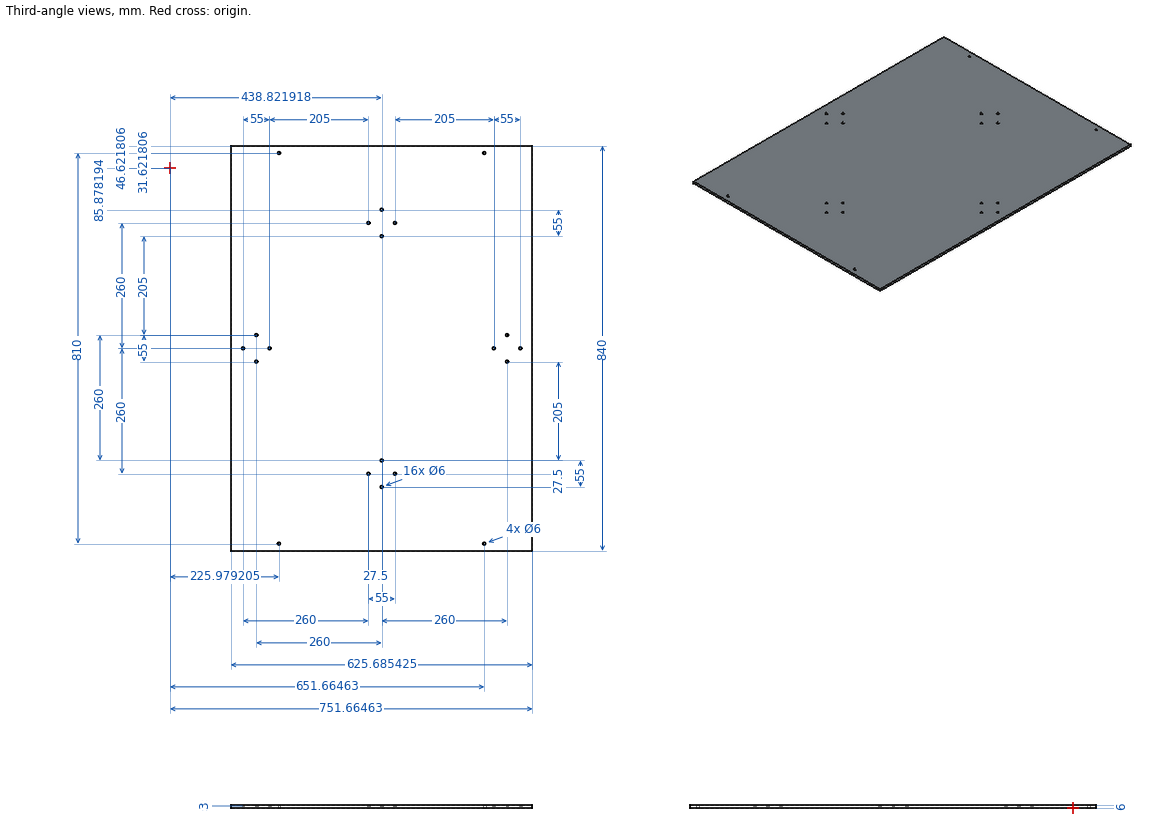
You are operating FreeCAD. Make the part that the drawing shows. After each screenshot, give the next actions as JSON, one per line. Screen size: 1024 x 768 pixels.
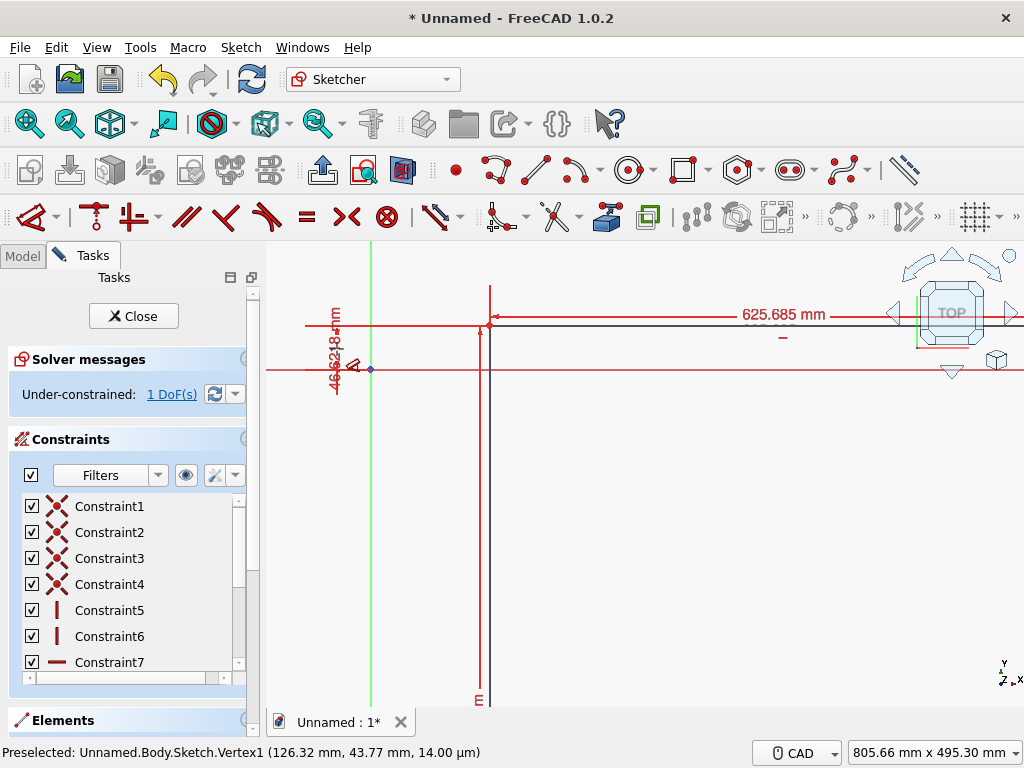
{"action": "scroll", "coordinate": [490, 330], "scroll_direction": "down", "scroll_amount": 5}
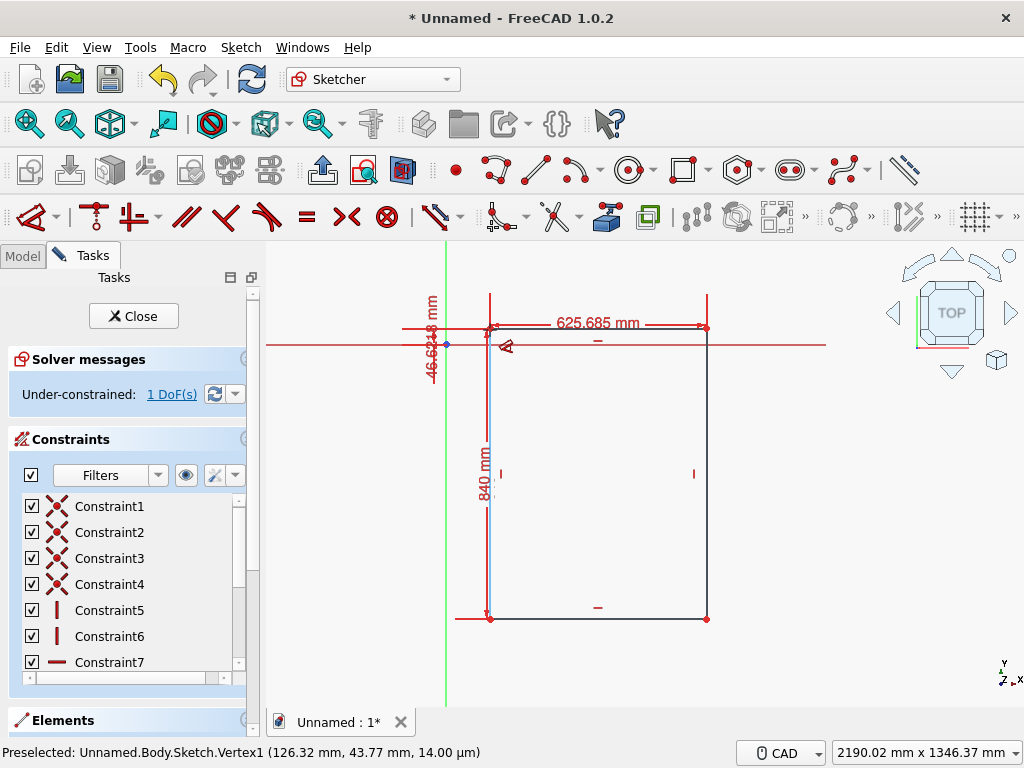
{"action": "left_click", "coordinate": [707, 619]}
{"action": "left_click", "coordinate": [576, 653]}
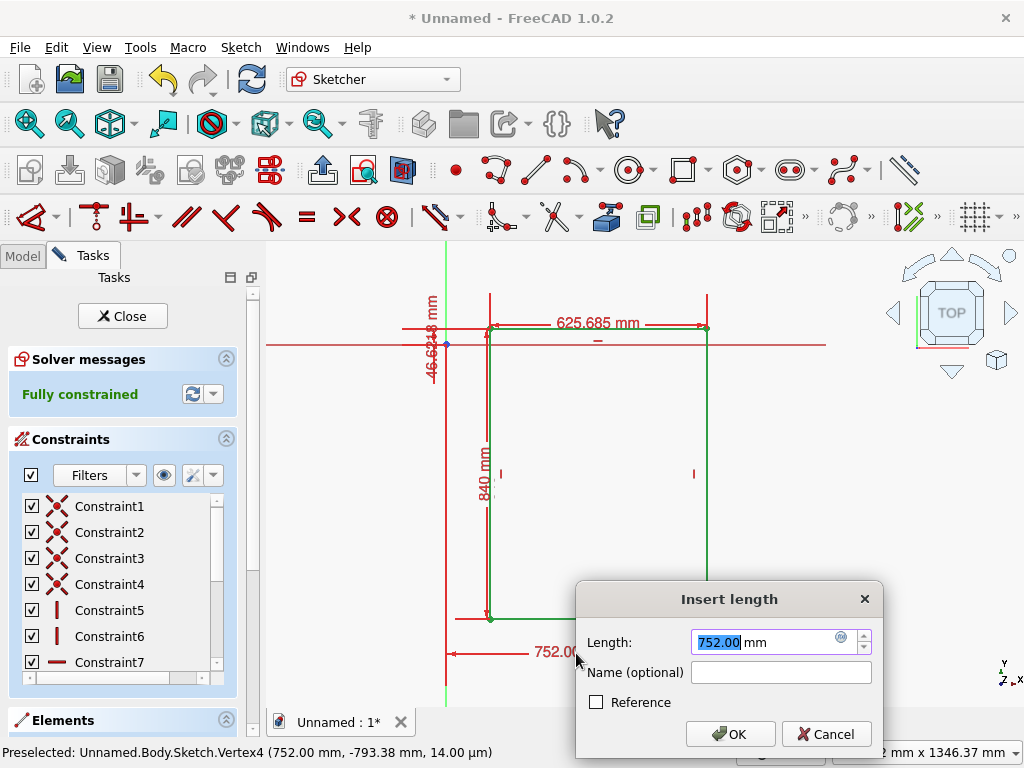
{"action": "type", "text": "751.66463"}
{"action": "key", "text": "Return"}
{"action": "key", "text": "Escape"}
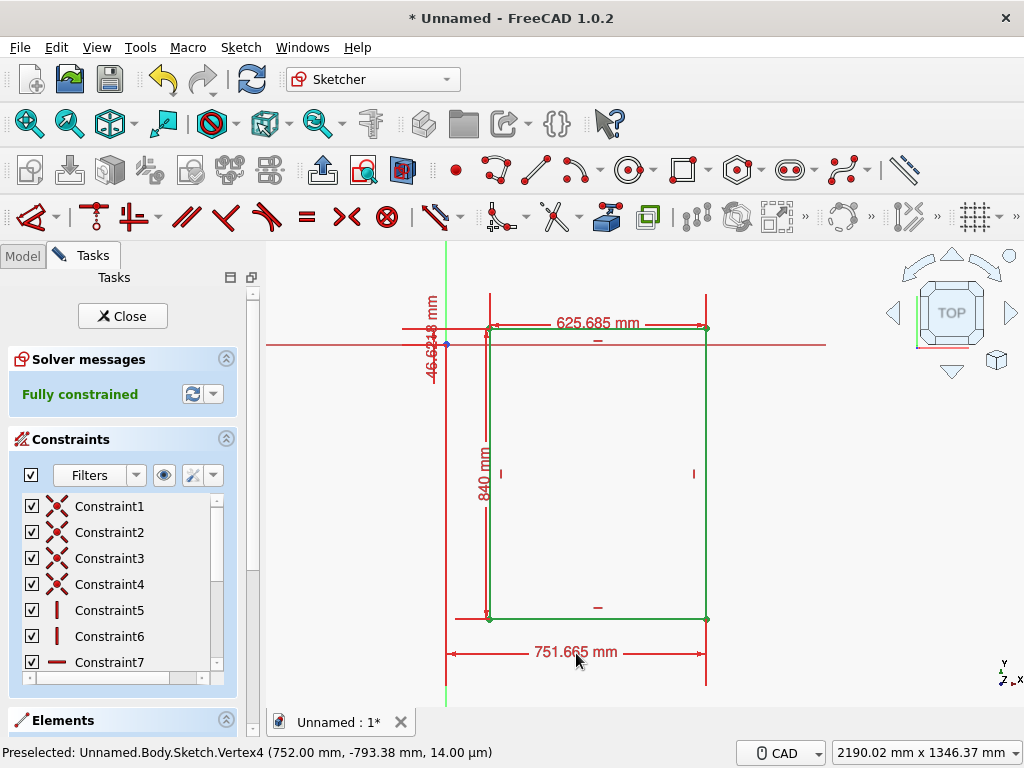
{"action": "left_click", "coordinate": [123, 316]}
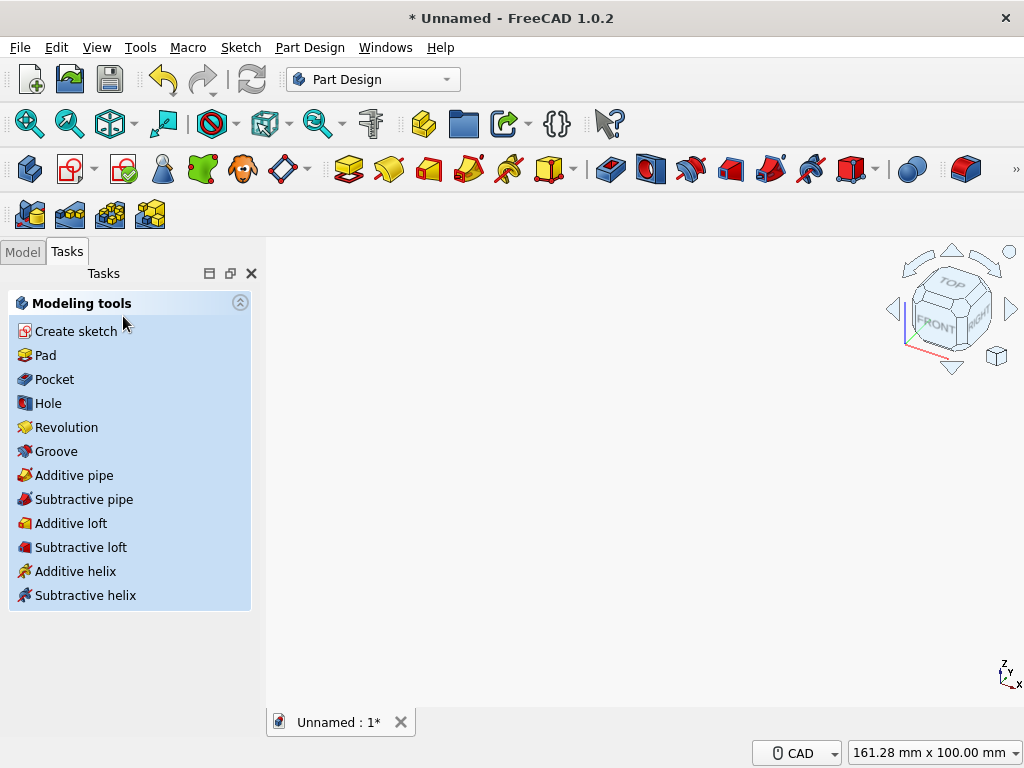
{"action": "left_click", "coordinate": [350, 170]}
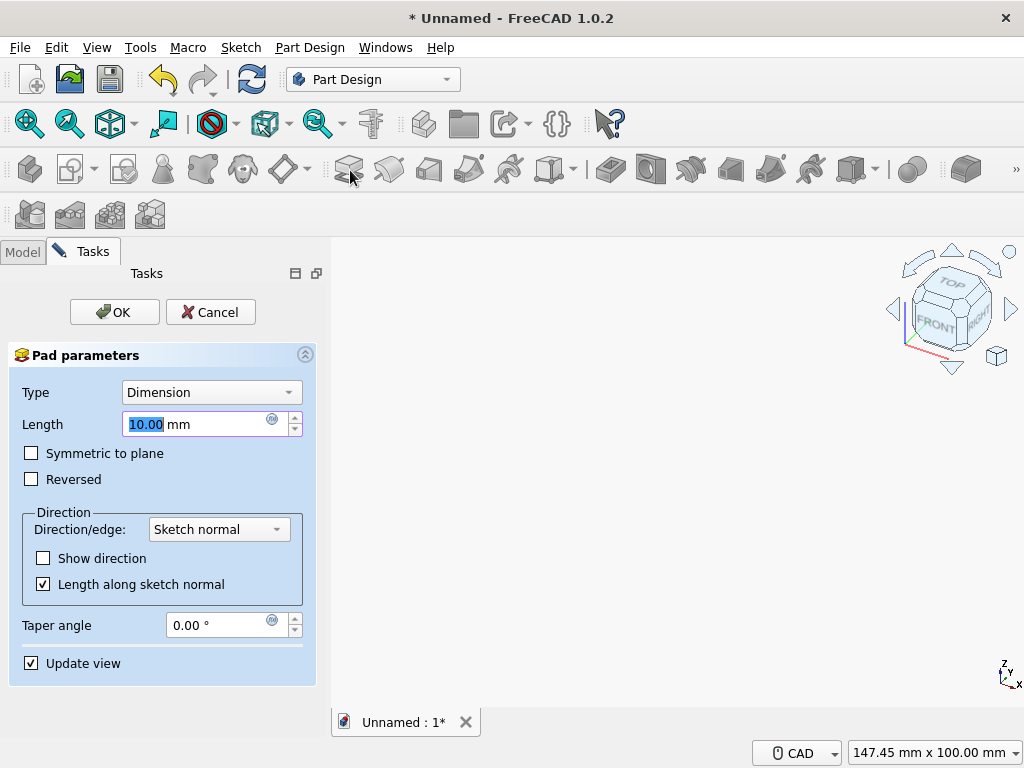
{"action": "type", "text": "6"}
{"action": "key", "text": "Tab"}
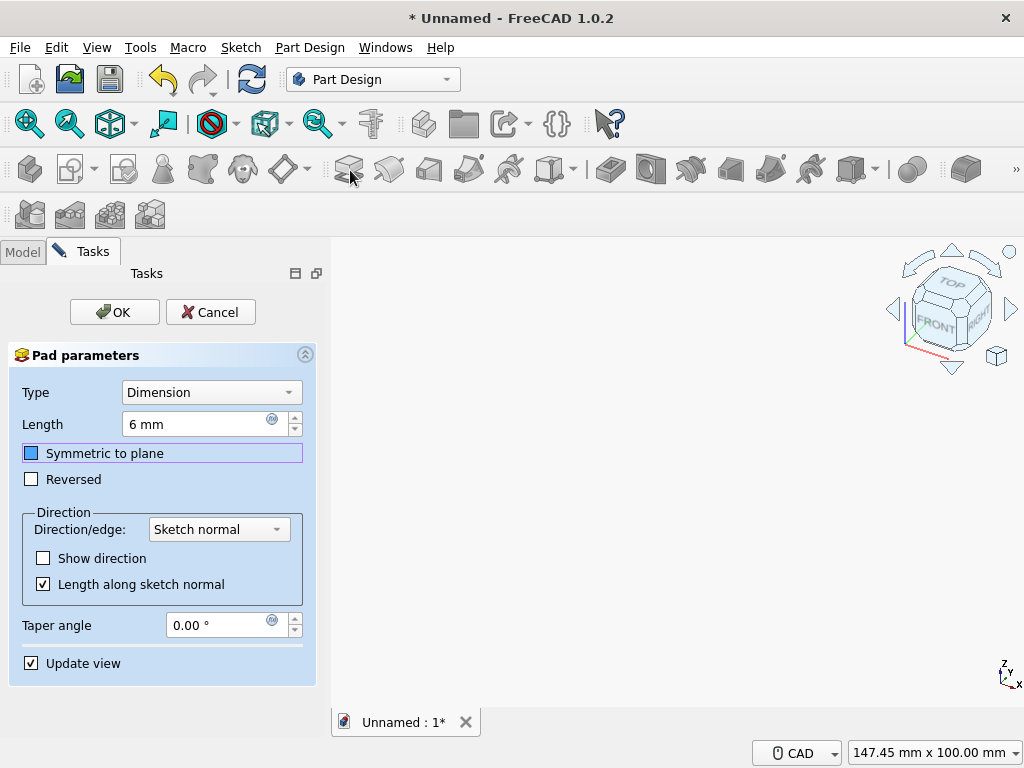
{"action": "left_click", "coordinate": [115, 312]}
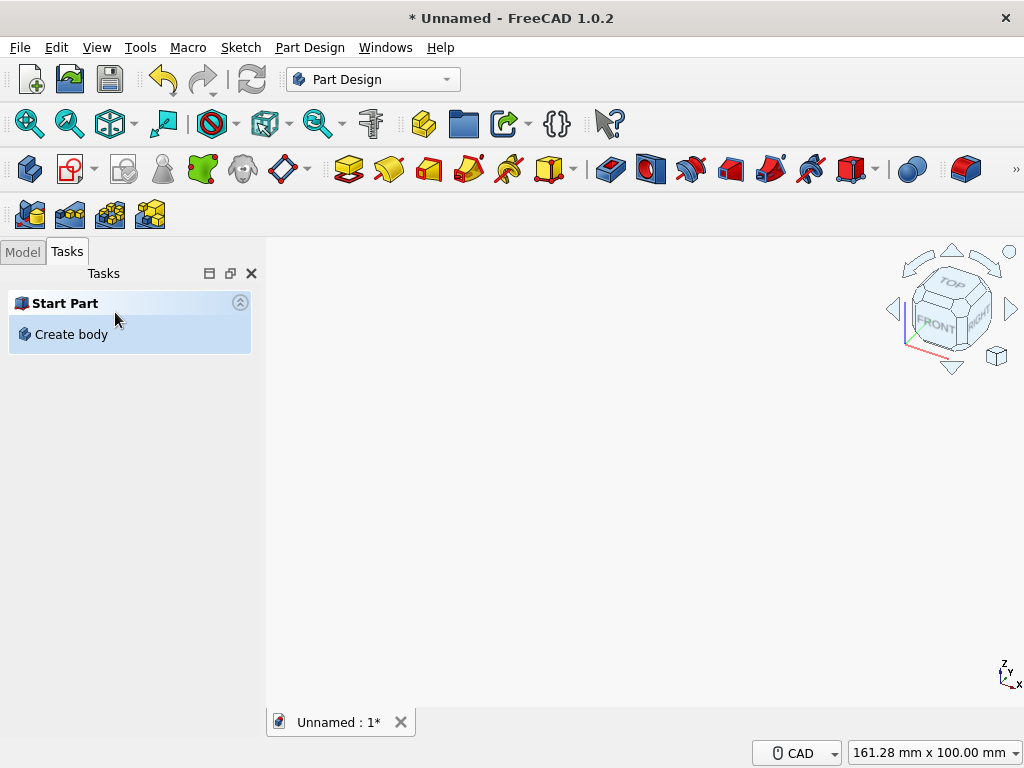
{"action": "left_click", "coordinate": [30, 124]}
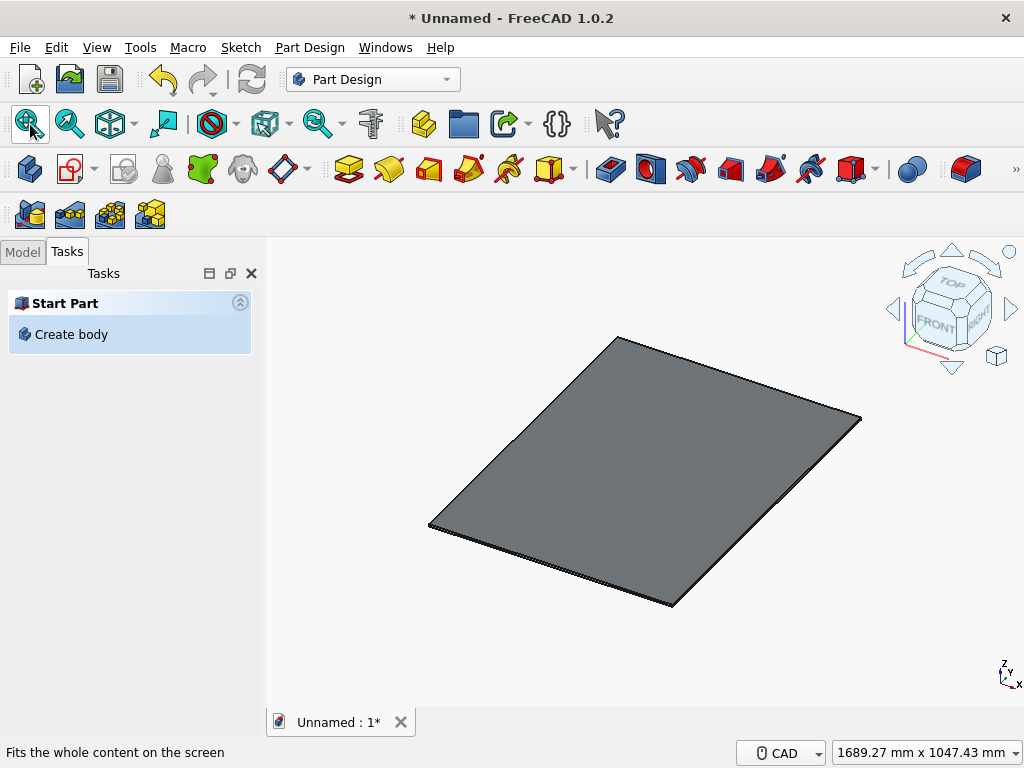
{"action": "left_click", "coordinate": [645, 470]}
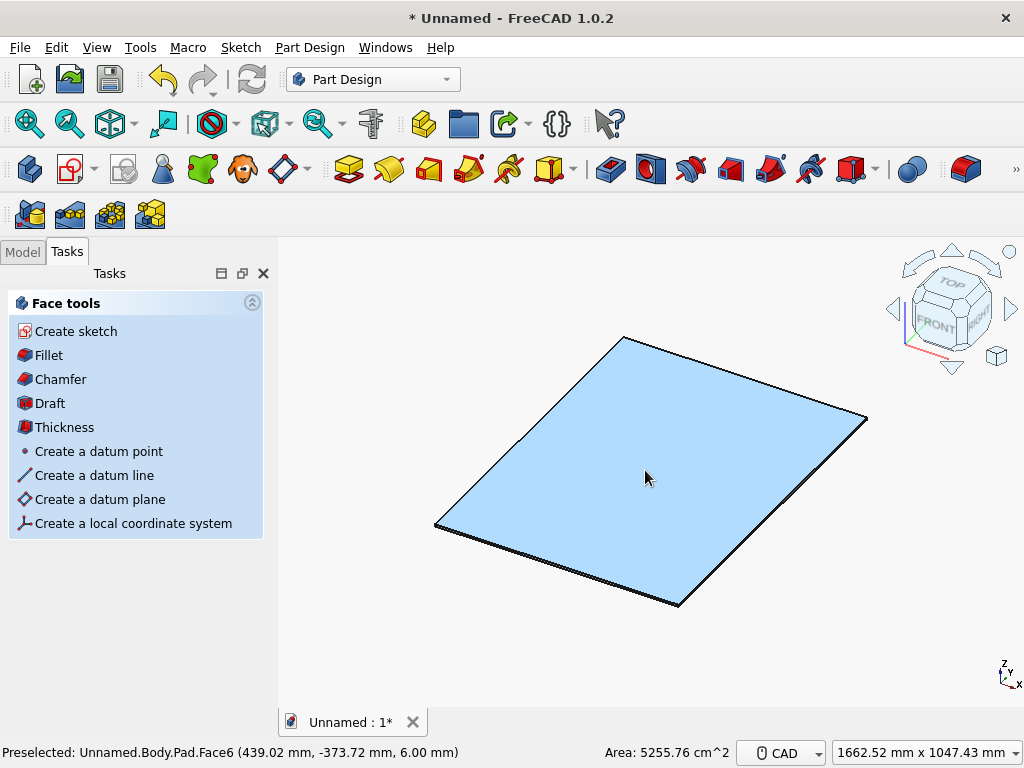
{"action": "left_click", "coordinate": [70, 170]}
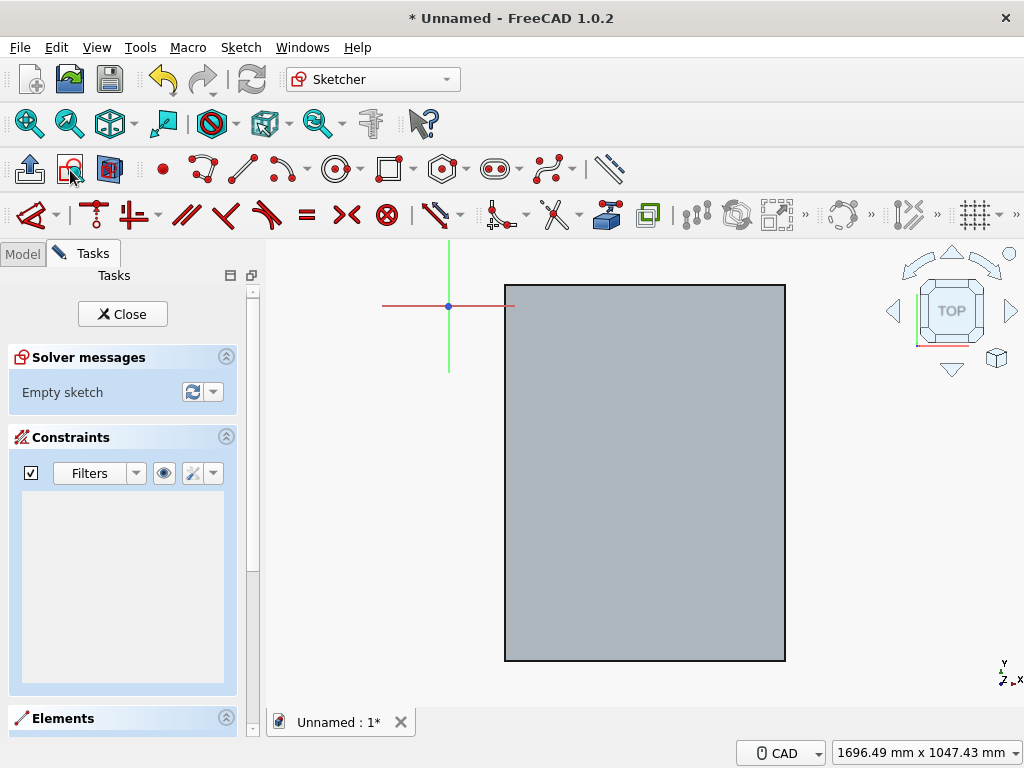
{"action": "left_click", "coordinate": [336, 170]}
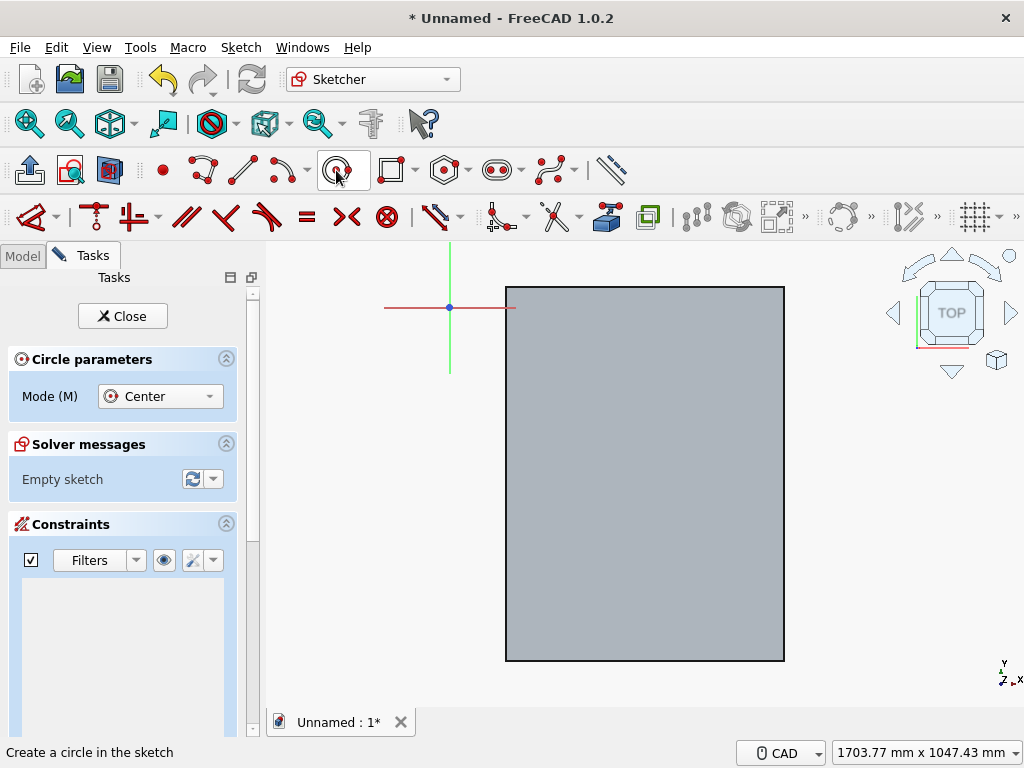
{"action": "scroll", "coordinate": [645, 602], "scroll_direction": "up", "scroll_amount": 15}